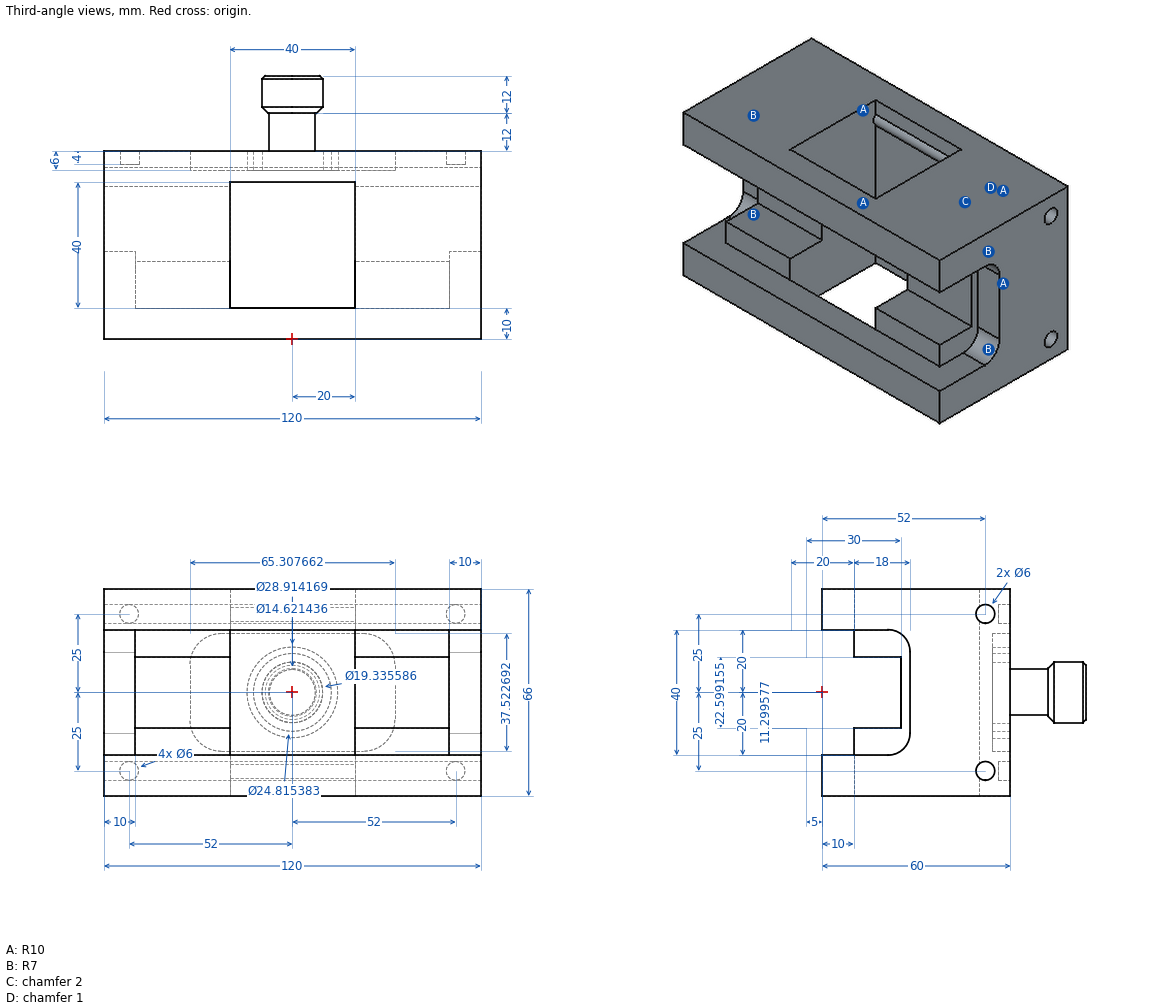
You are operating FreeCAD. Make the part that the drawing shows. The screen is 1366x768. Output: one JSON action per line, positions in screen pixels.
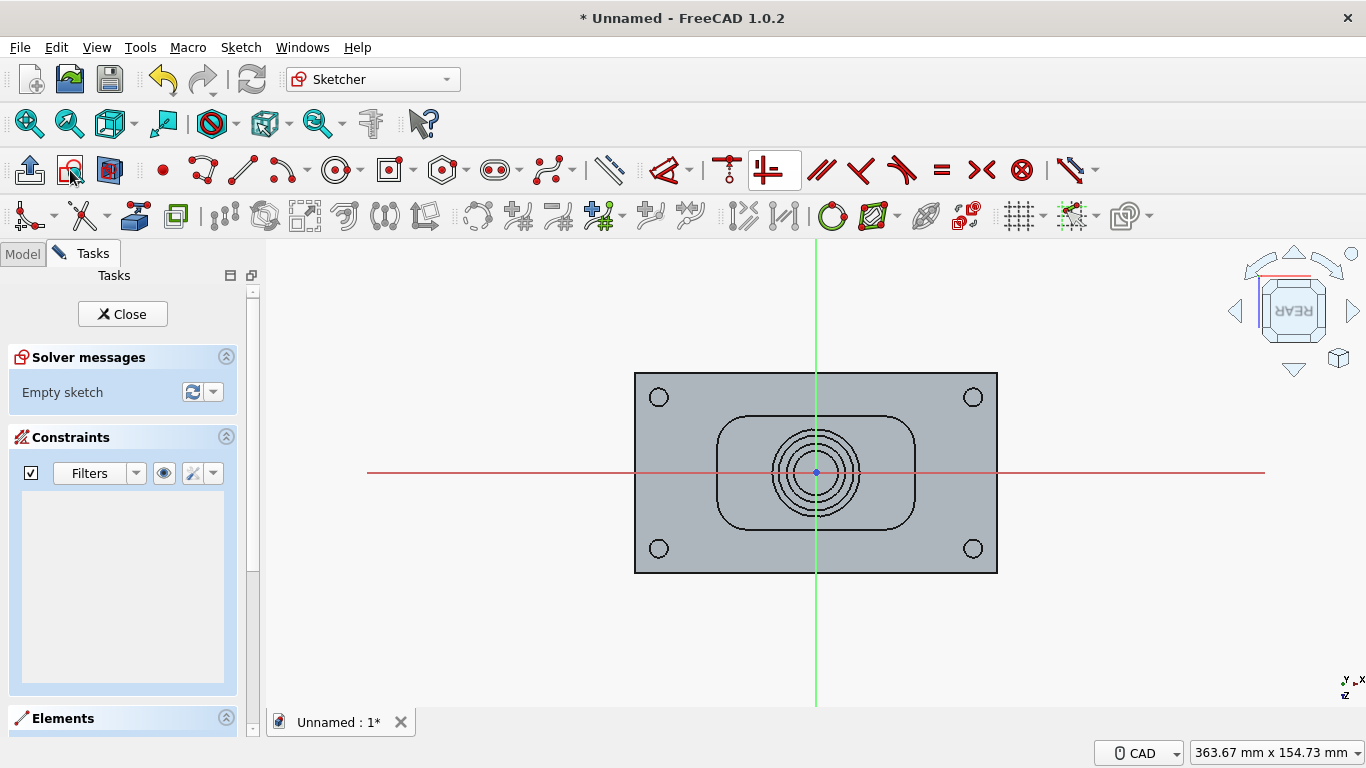
{"action": "scroll", "coordinate": [833, 473], "scroll_direction": "up", "scroll_amount": 8}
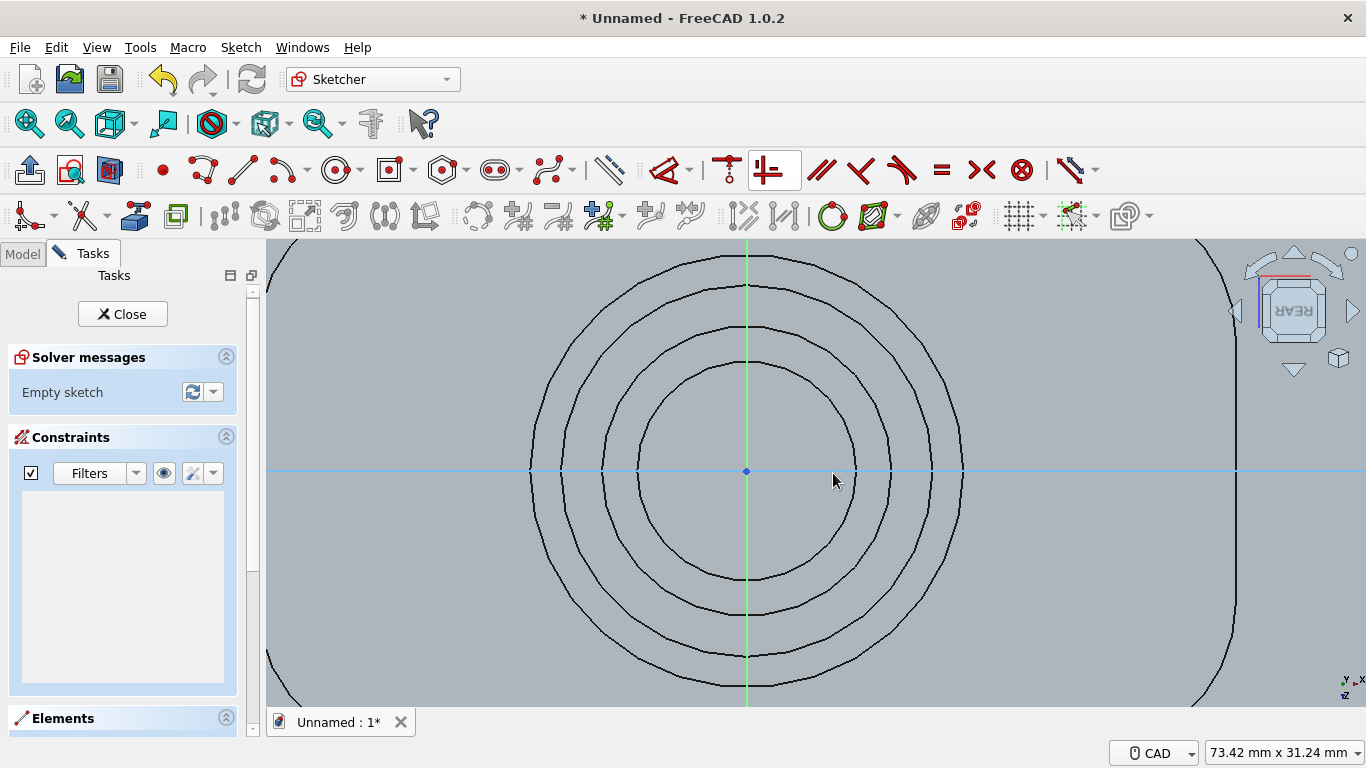
{"action": "left_click", "coordinate": [336, 170]}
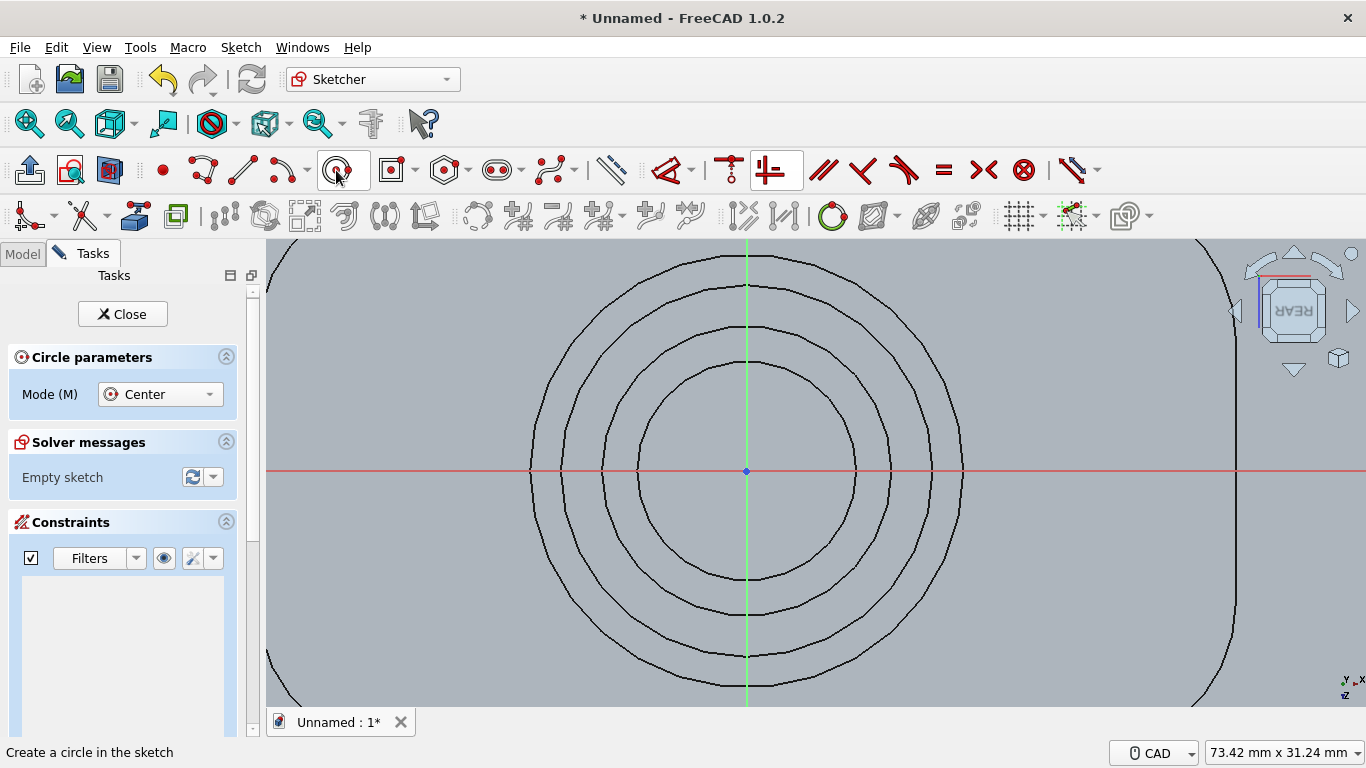
{"action": "left_click", "coordinate": [747, 471]}
{"action": "mouse_move", "coordinate": [849, 369]}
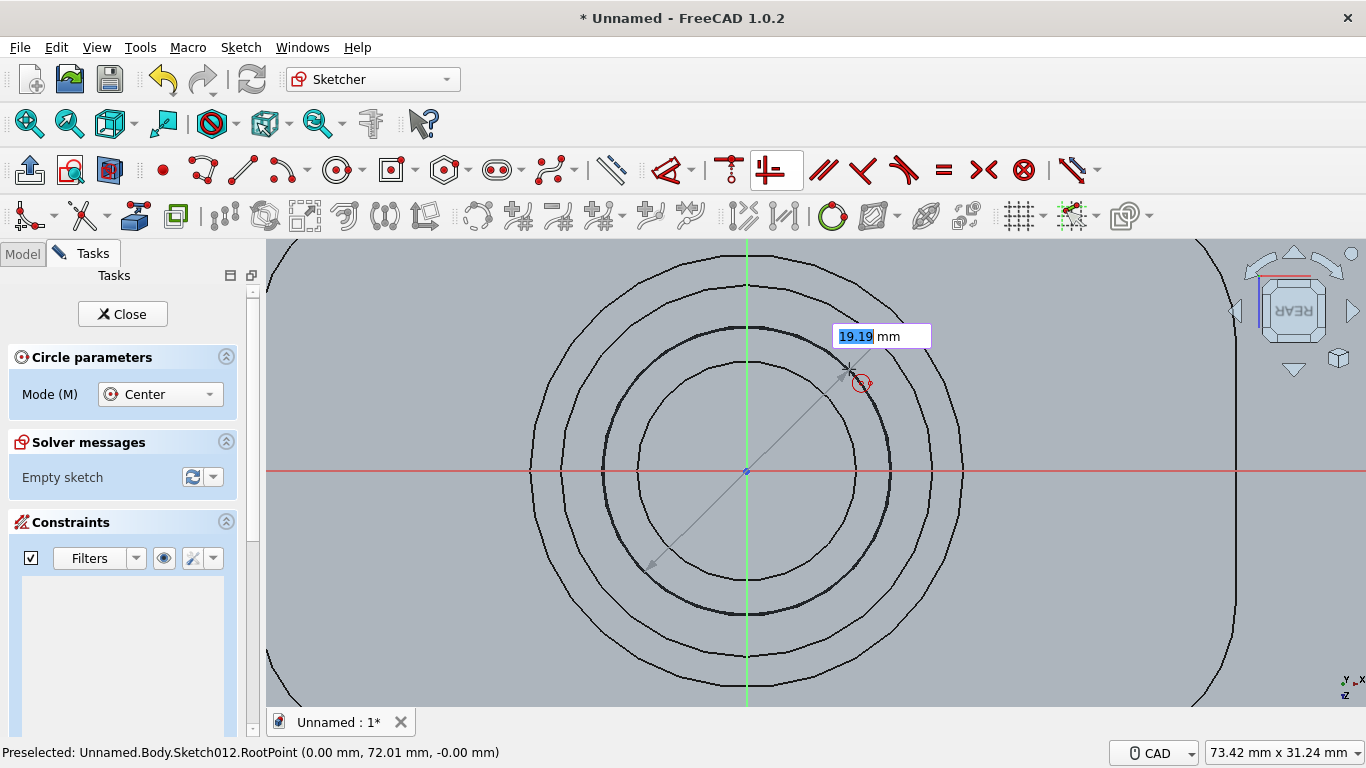
{"action": "type", "text": "19.335586"}
{"action": "key", "text": "Return"}
{"action": "key", "text": "Escape"}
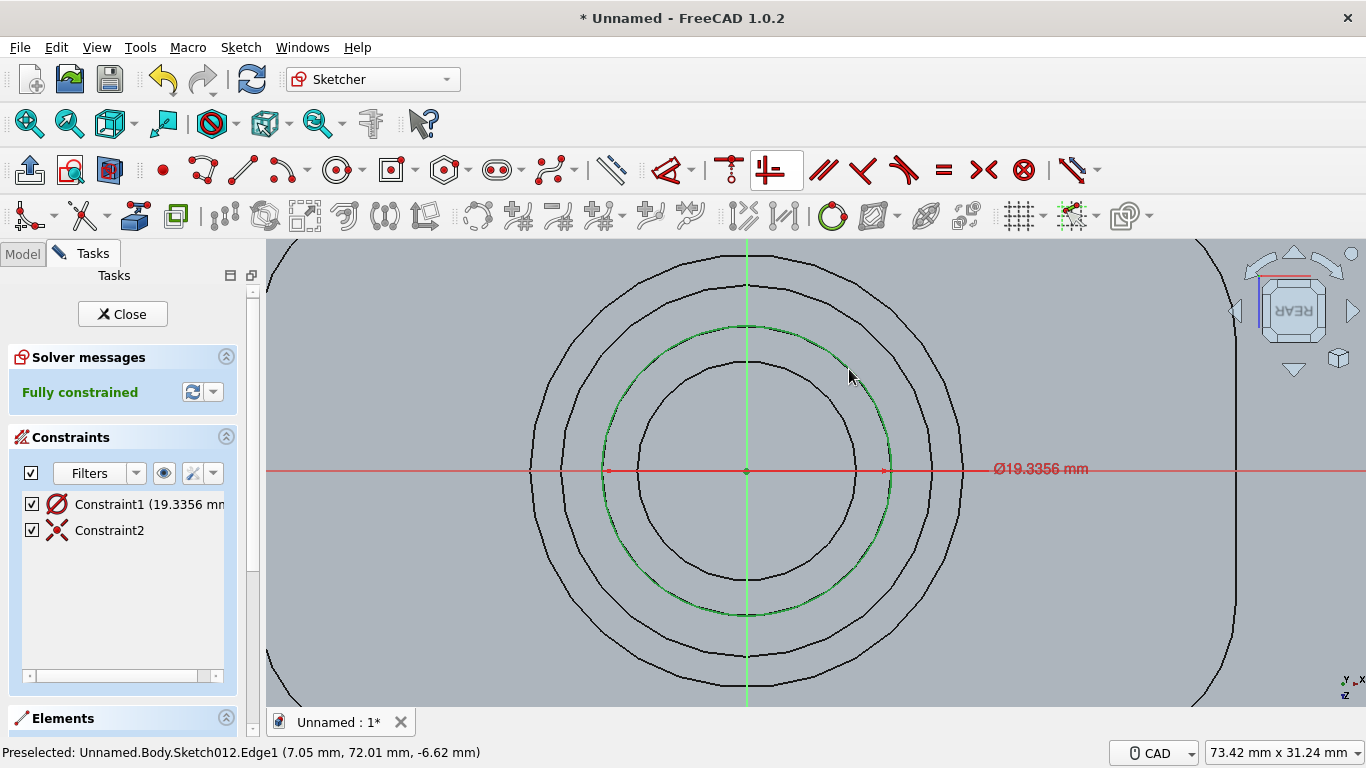
{"action": "left_click", "coordinate": [123, 314]}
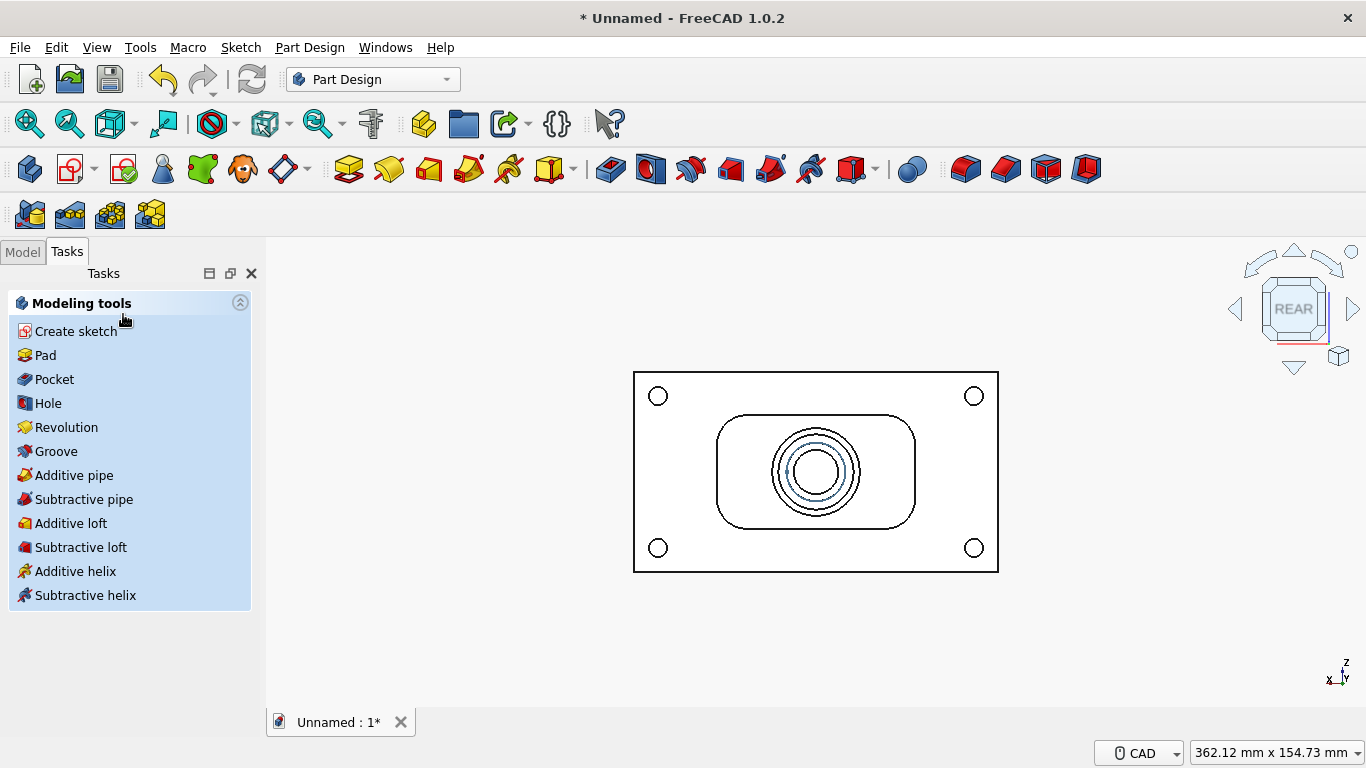
{"action": "left_click", "coordinate": [350, 170]}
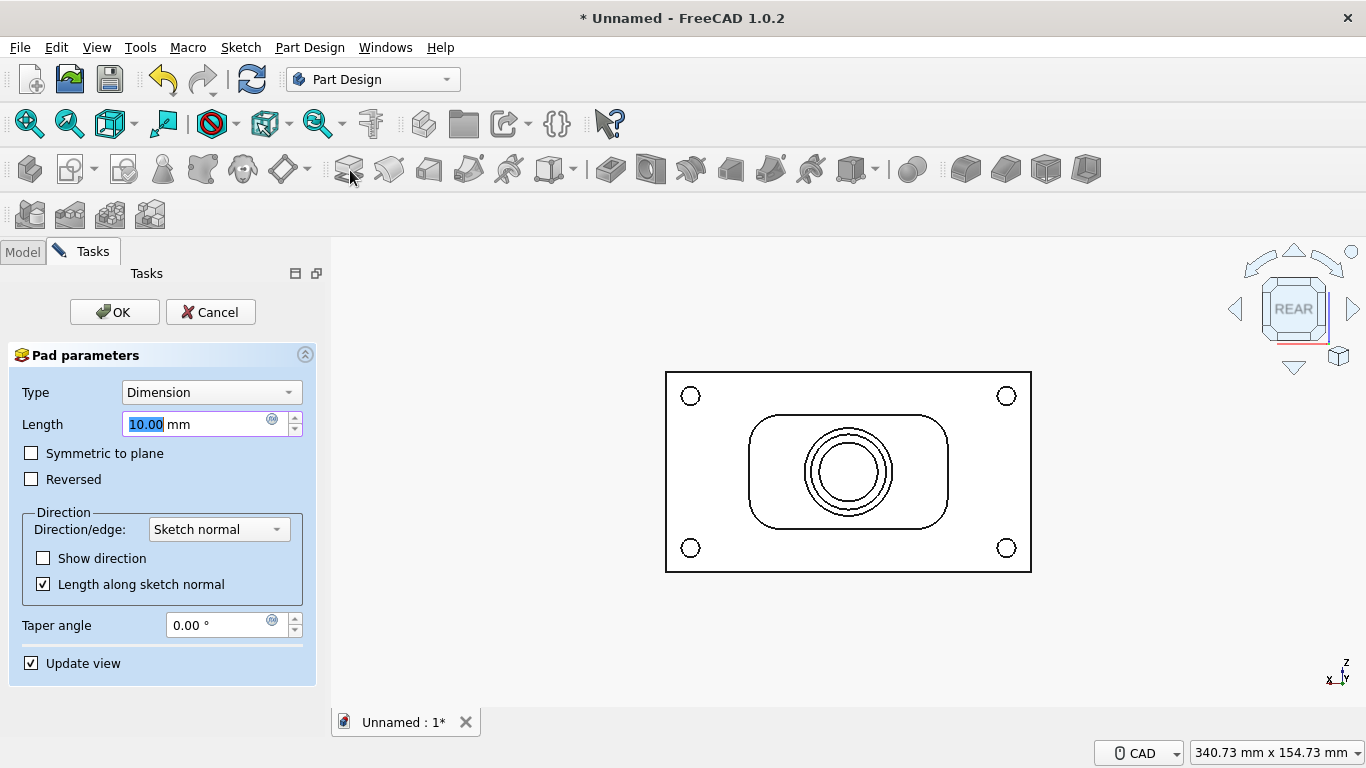
{"action": "type", "text": "12"}
{"action": "key", "text": "Tab"}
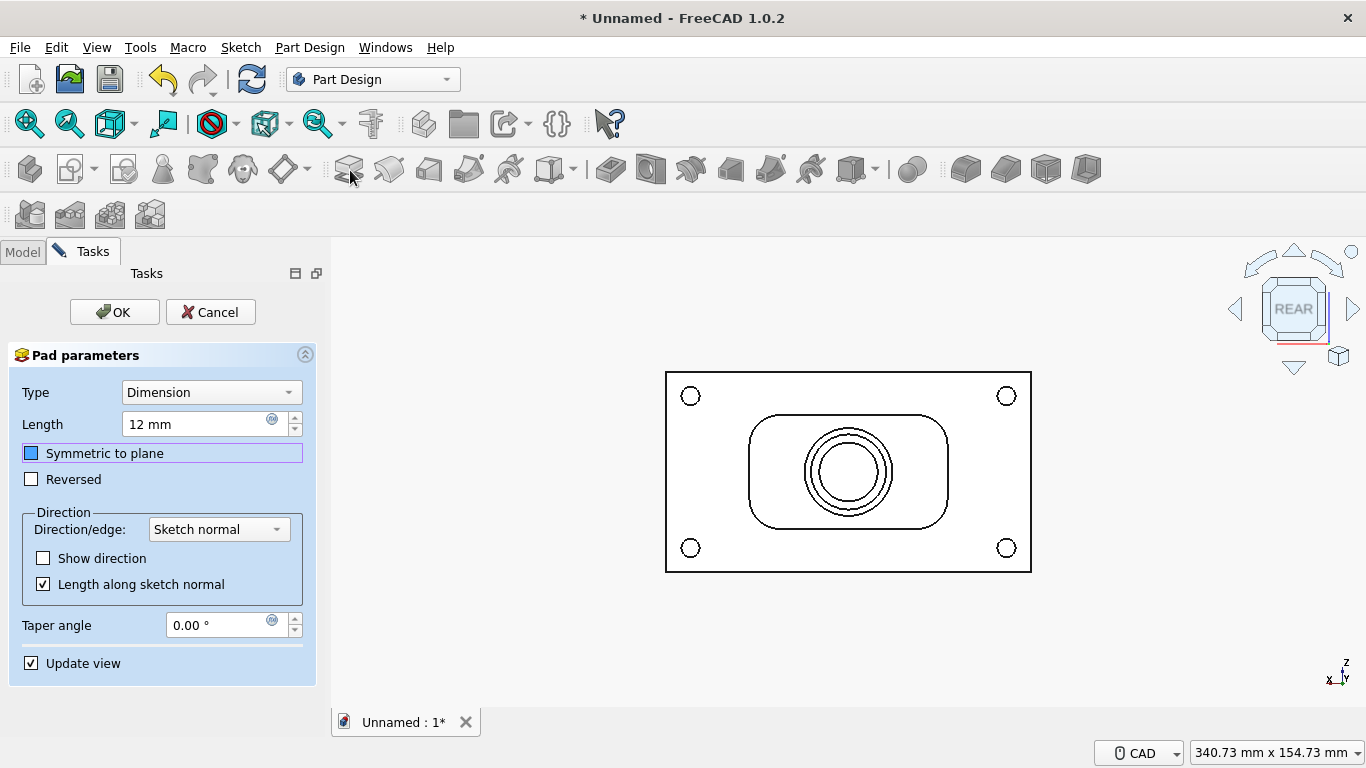
{"action": "left_click", "coordinate": [115, 312]}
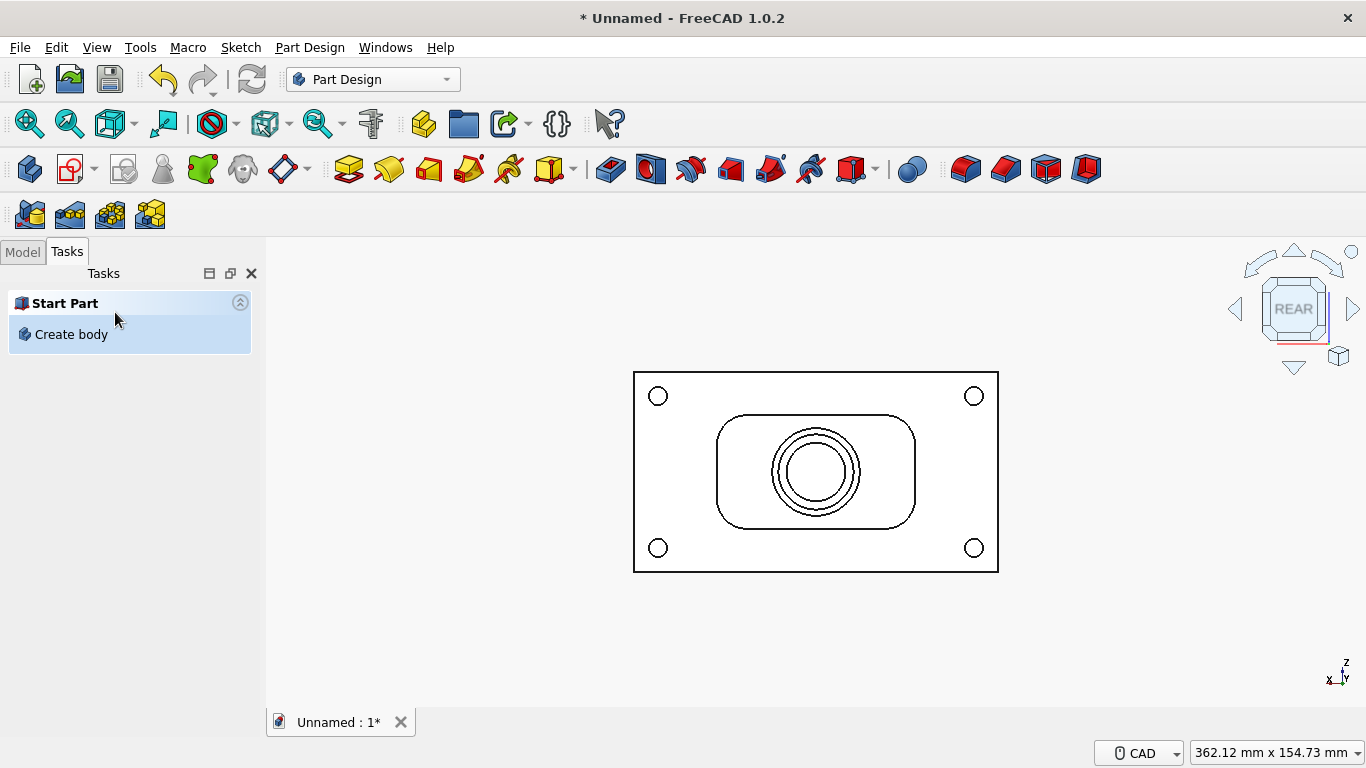
{"action": "left_click", "coordinate": [30, 124]}